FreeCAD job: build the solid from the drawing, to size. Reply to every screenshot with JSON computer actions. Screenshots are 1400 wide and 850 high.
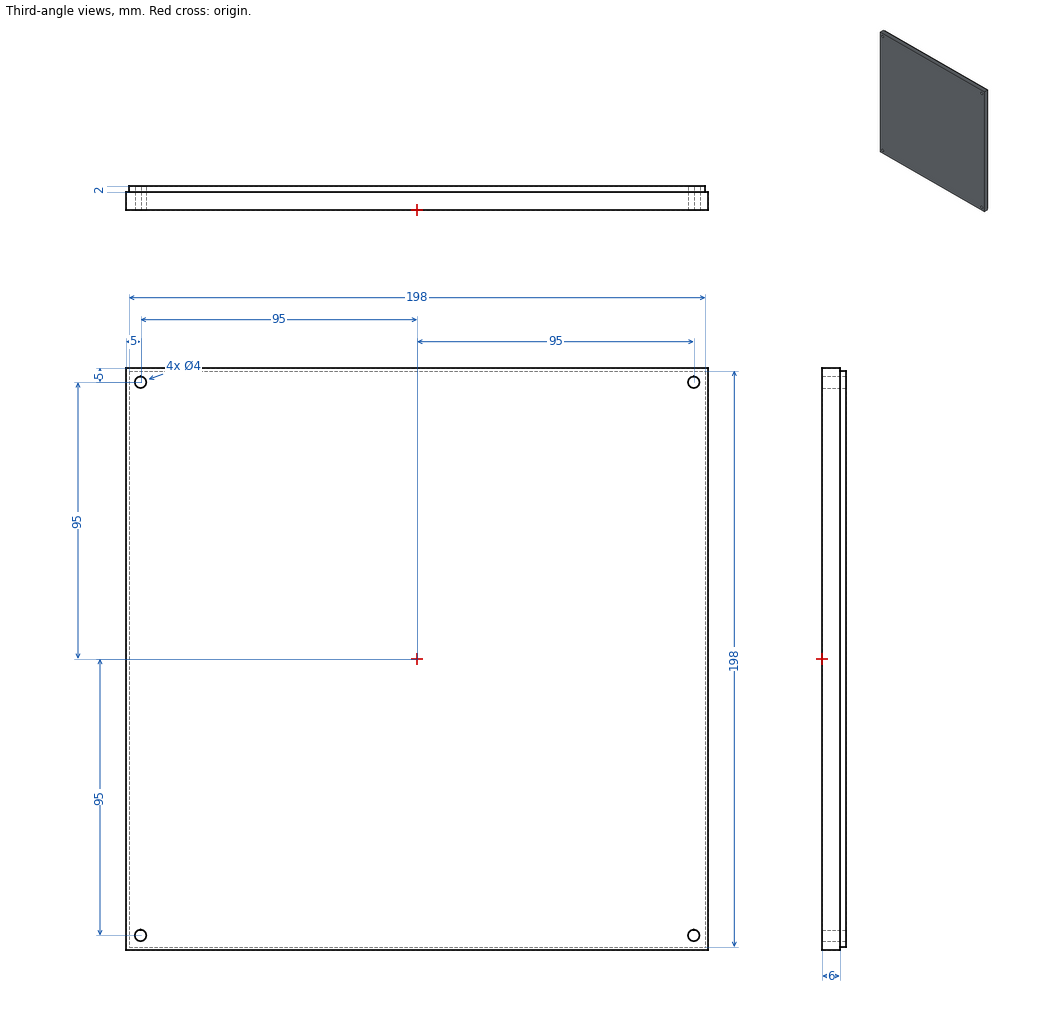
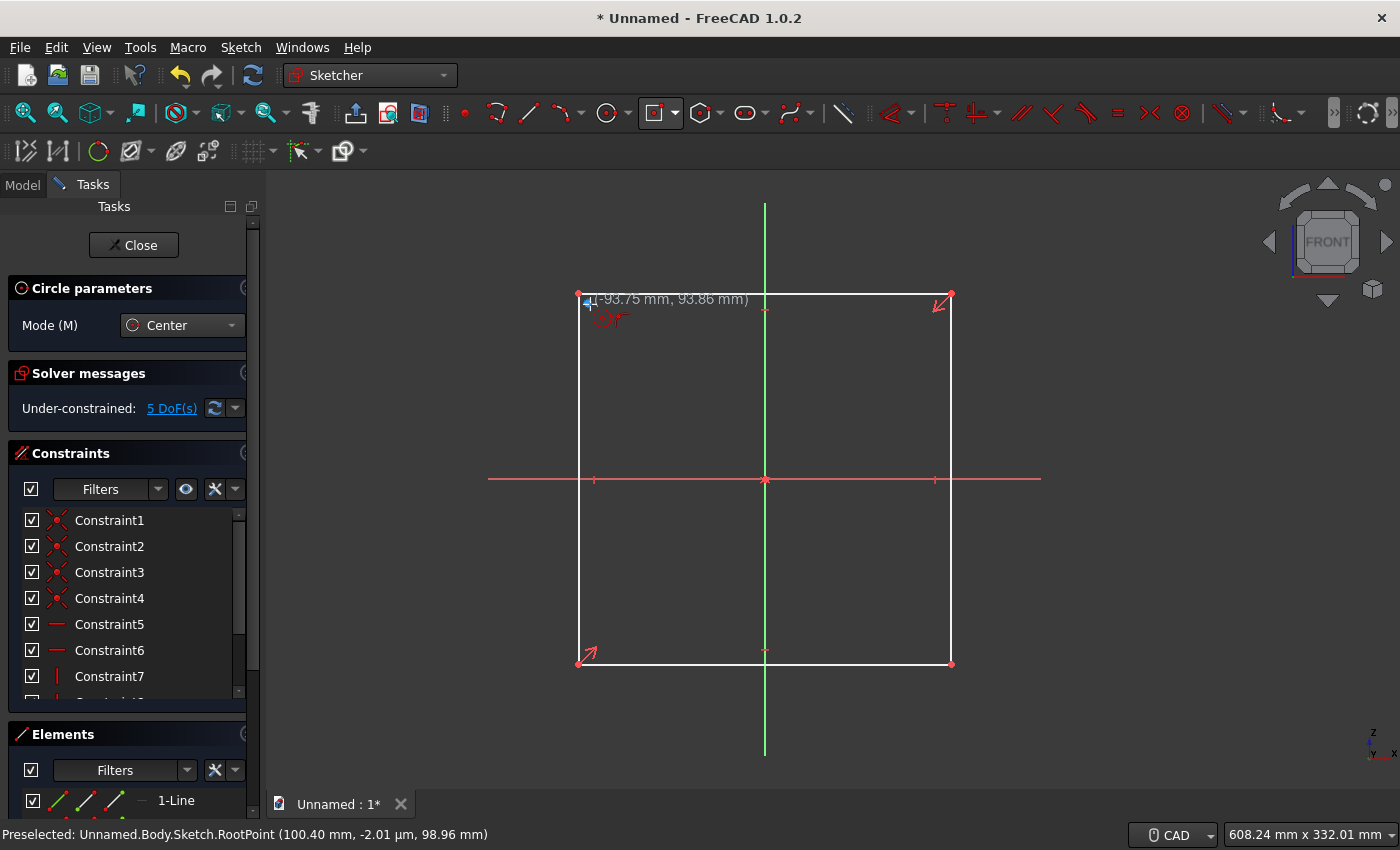
{"action": "scroll", "coordinate": [942, 302], "scroll_direction": "up", "scroll_amount": 10}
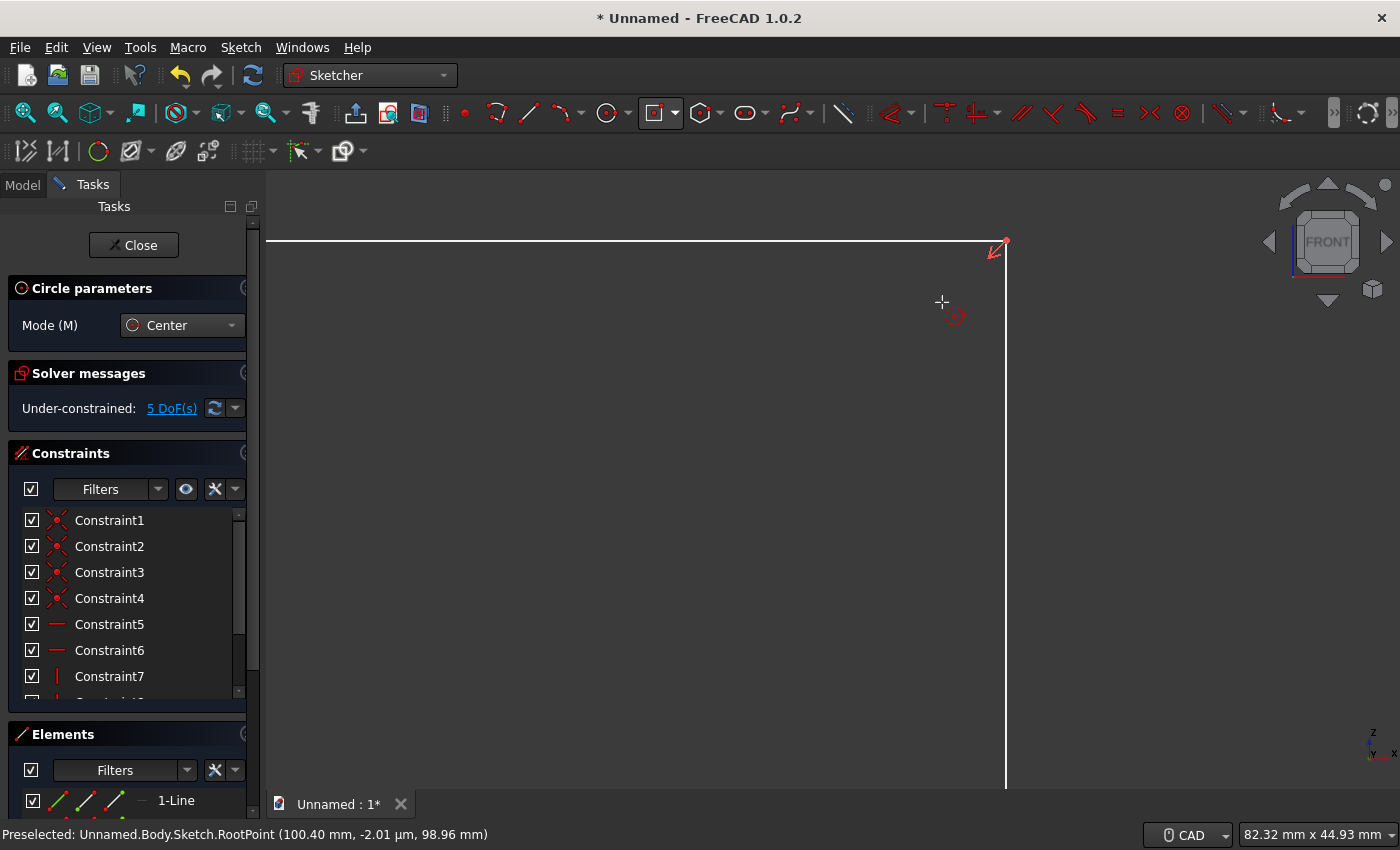
{"action": "scroll", "coordinate": [942, 302], "scroll_direction": "down", "scroll_amount": 10}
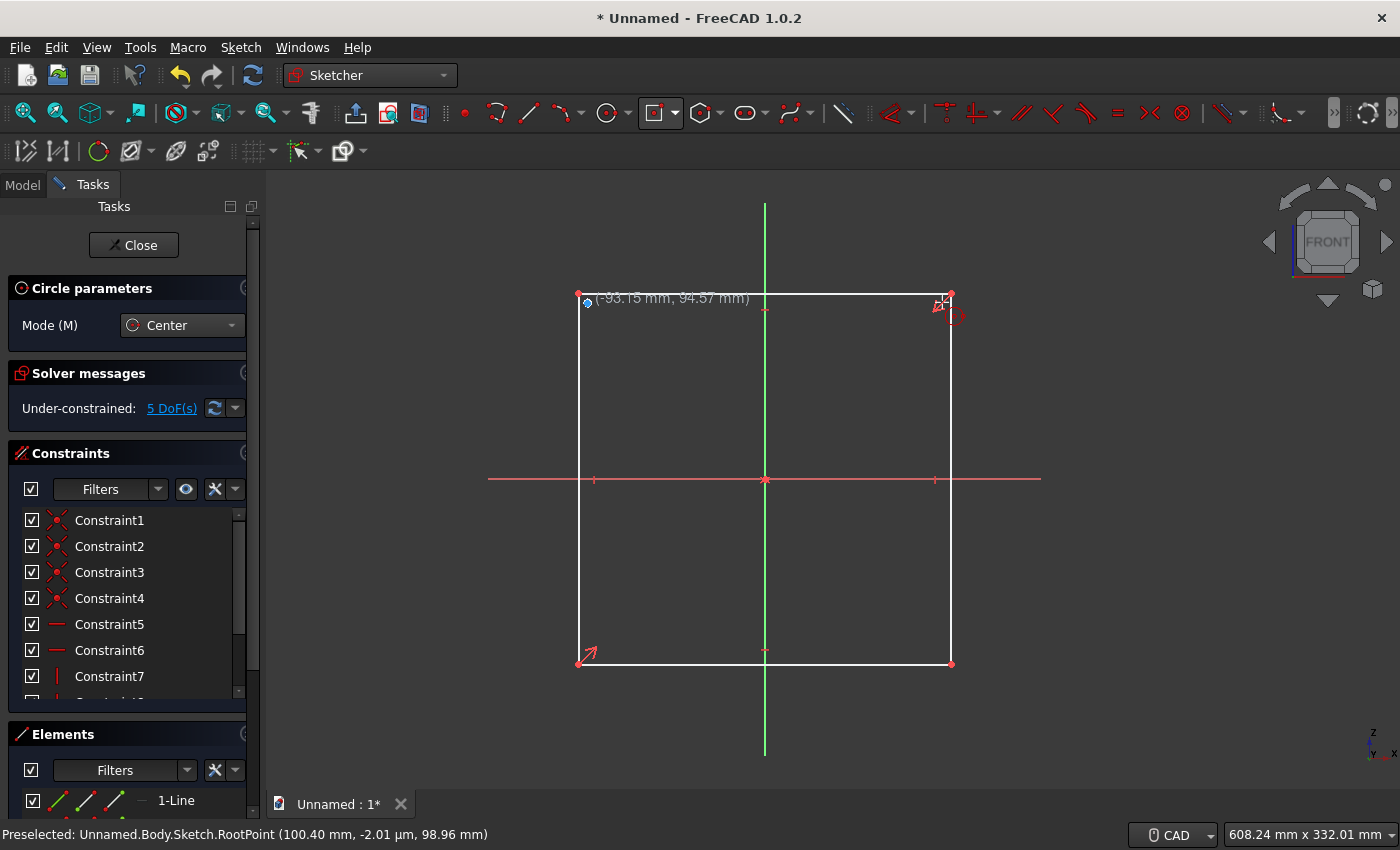
{"action": "scroll", "coordinate": [942, 302], "scroll_direction": "up", "scroll_amount": 3}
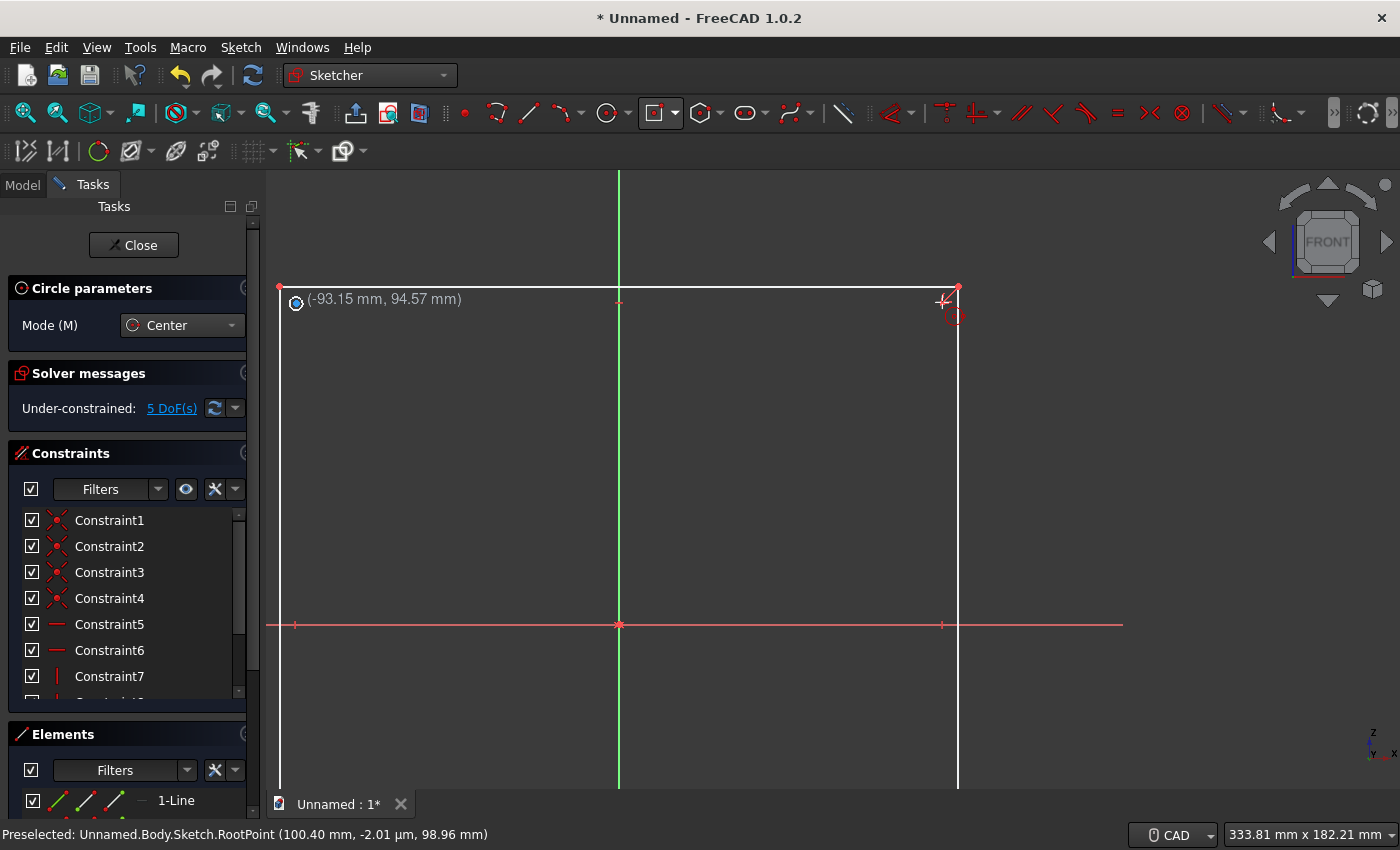
{"action": "left_click", "coordinate": [942, 302]}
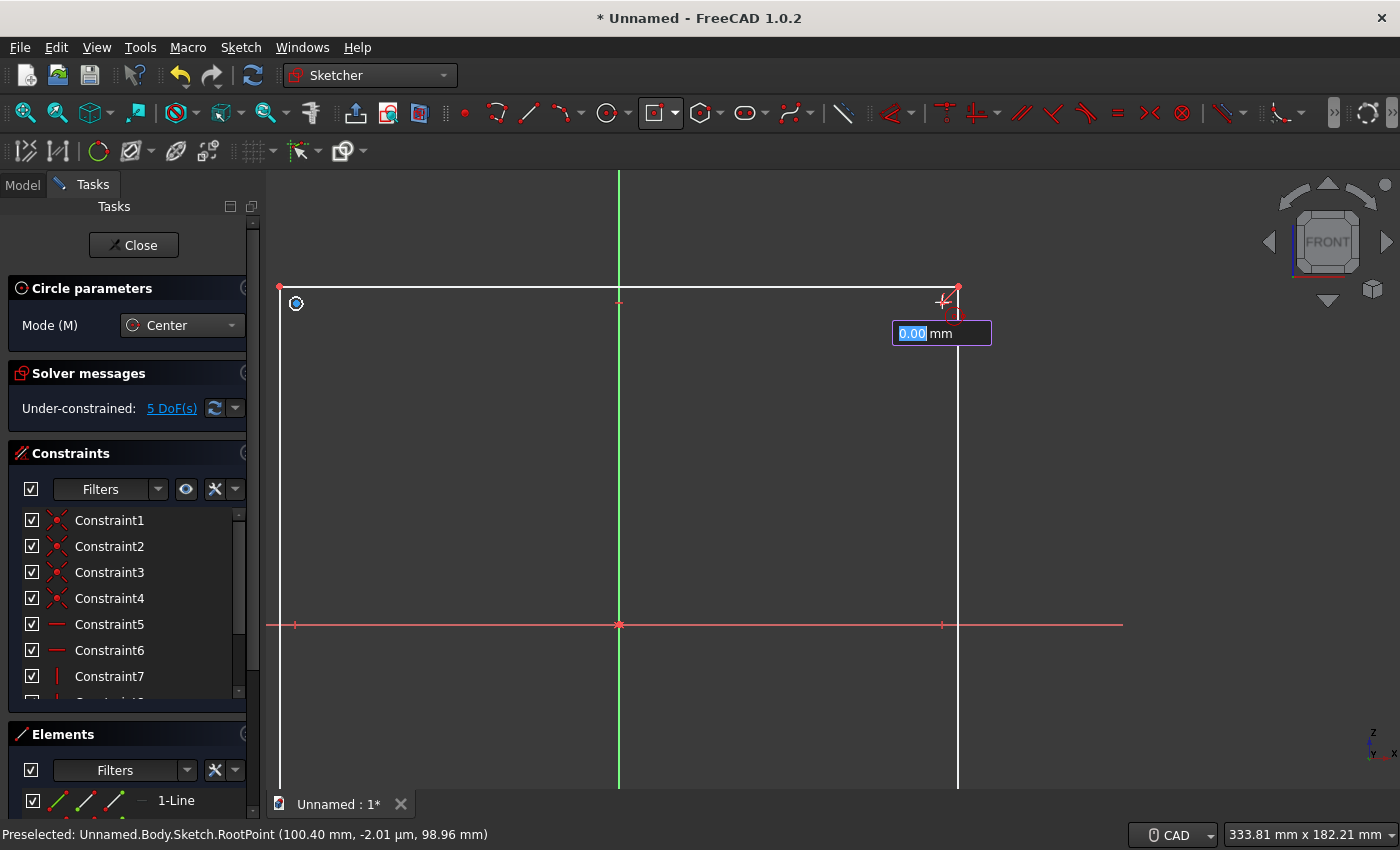
{"action": "scroll", "coordinate": [937, 307], "scroll_direction": "up", "scroll_amount": 5}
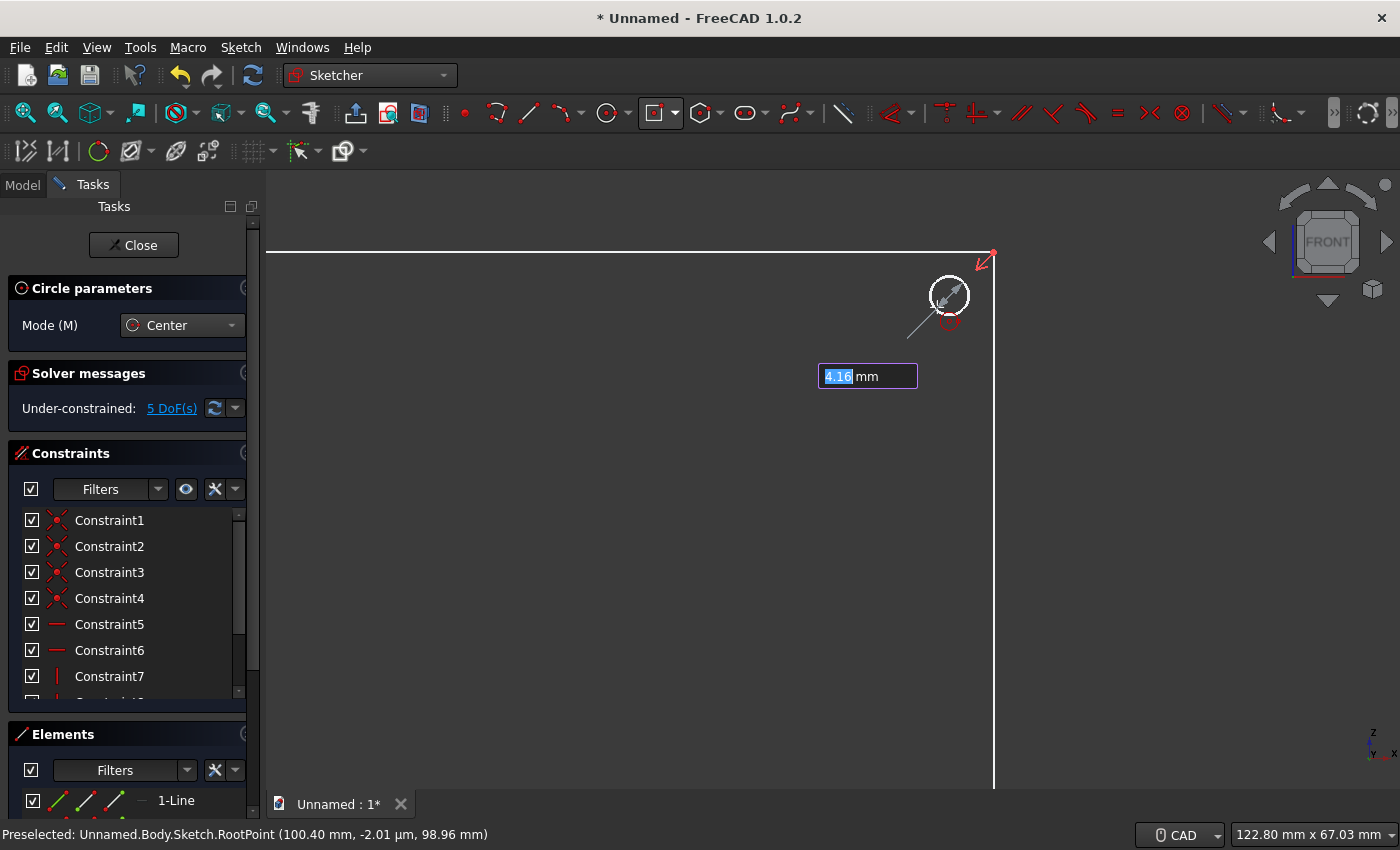
{"action": "left_click", "coordinate": [936, 307]}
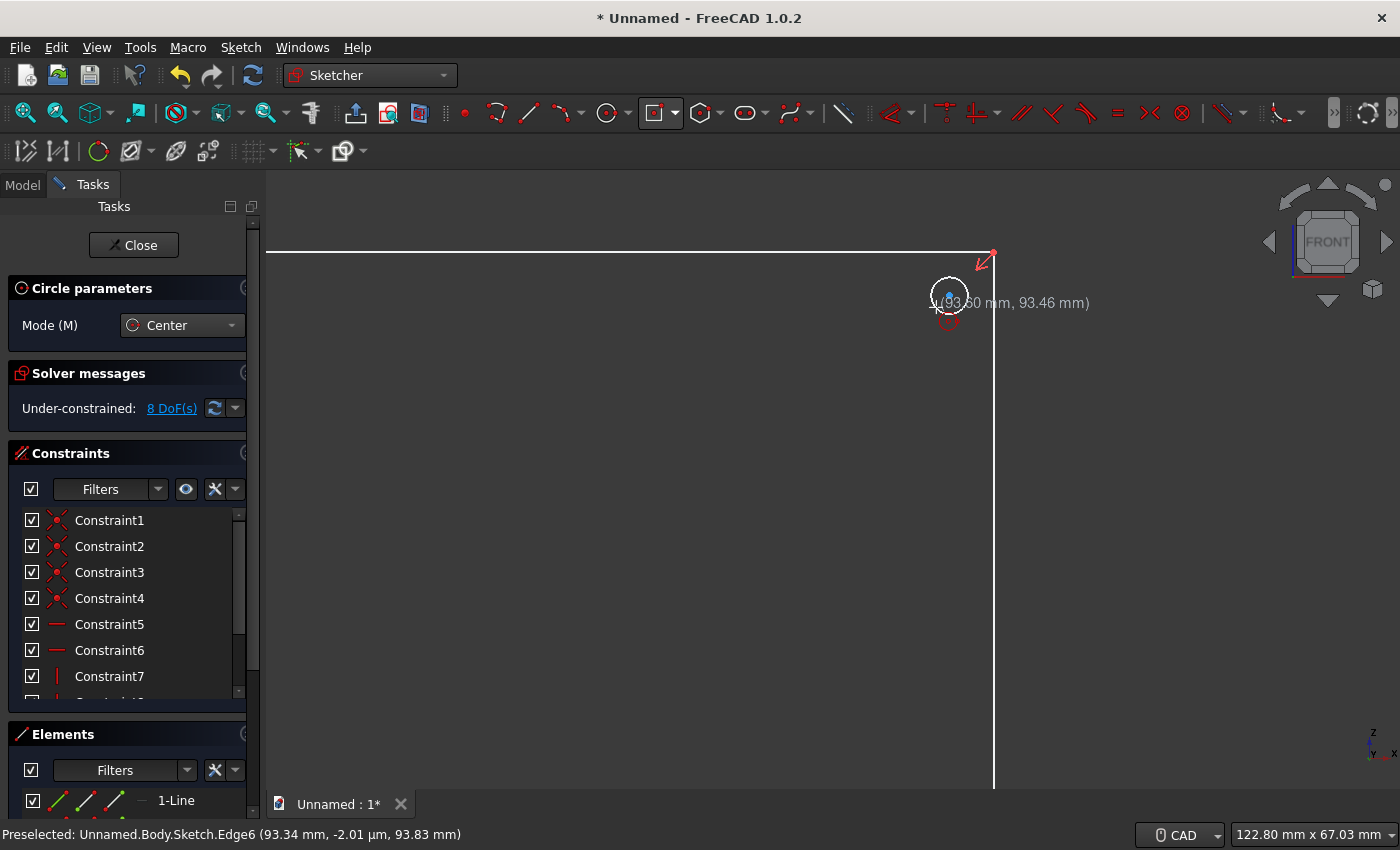
{"action": "scroll", "coordinate": [940, 305], "scroll_direction": "down", "scroll_amount": 8}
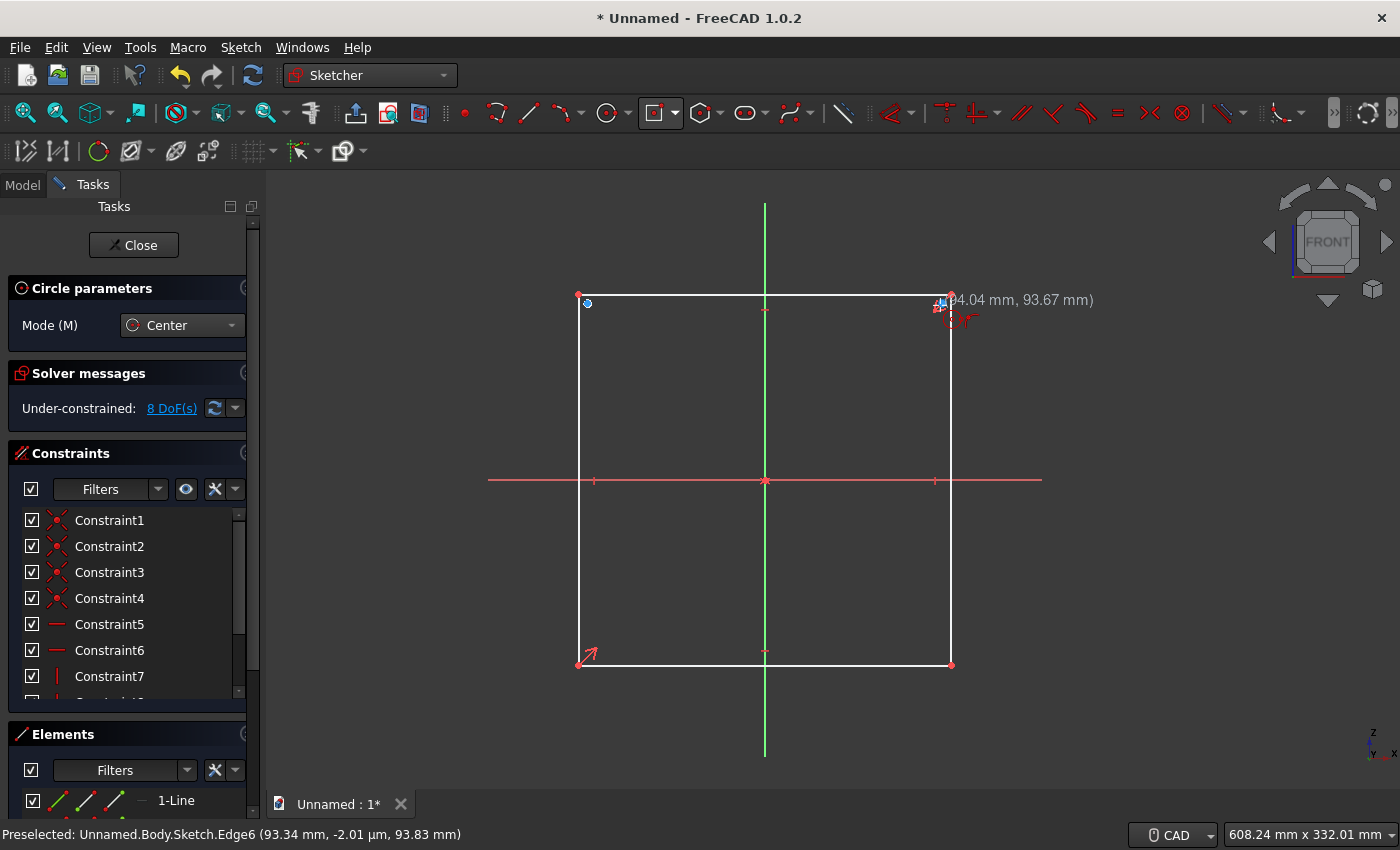
{"action": "scroll", "coordinate": [588, 657], "scroll_direction": "up", "scroll_amount": 10}